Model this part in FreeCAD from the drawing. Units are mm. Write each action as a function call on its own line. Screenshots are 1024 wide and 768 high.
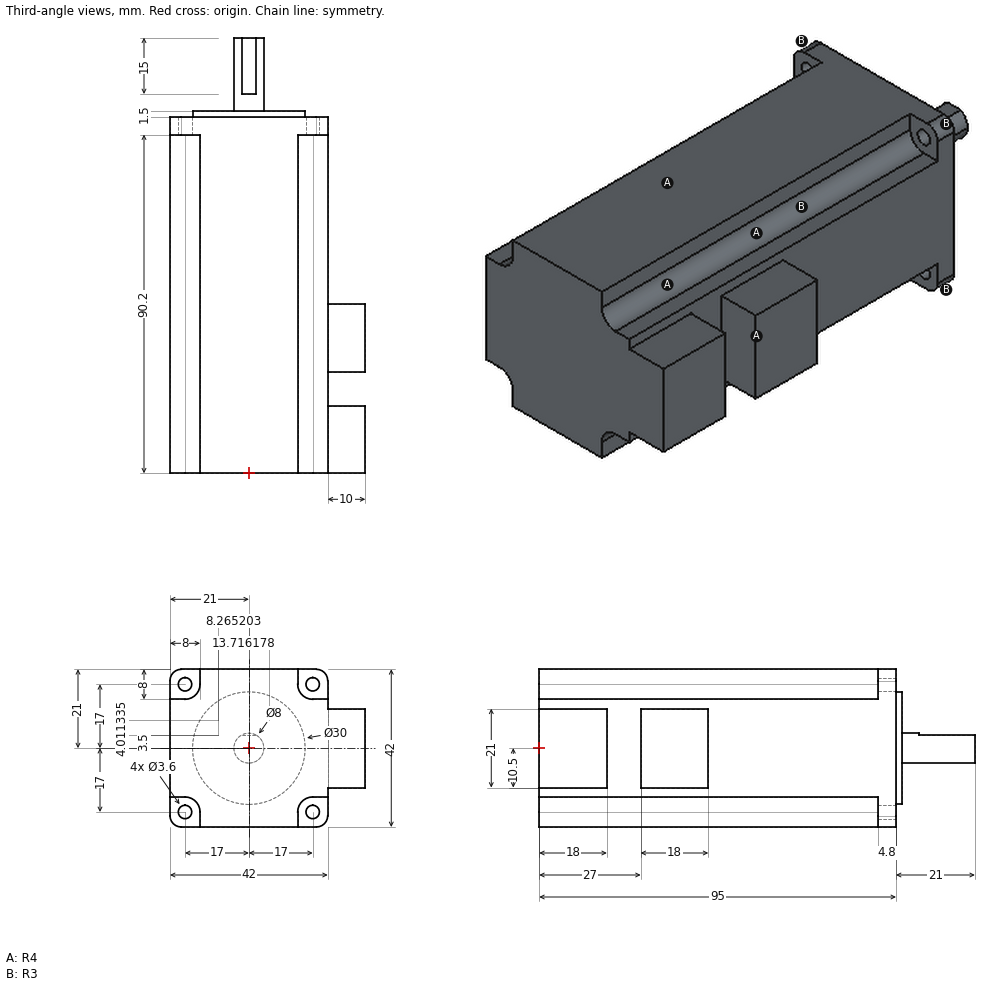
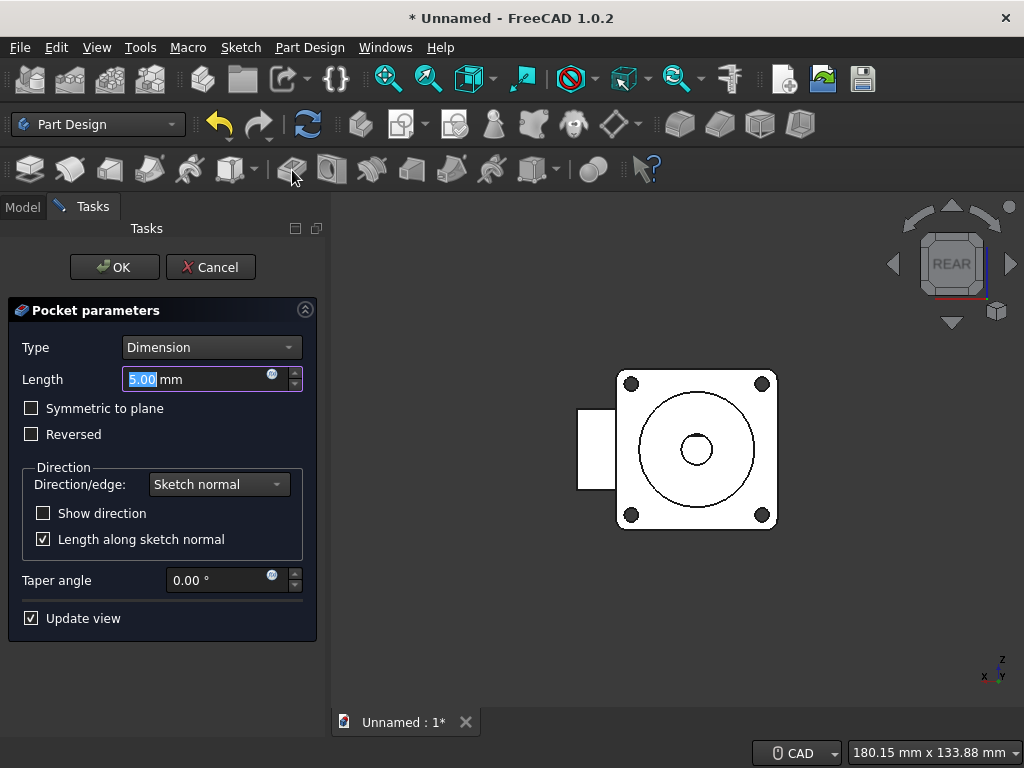
text(15)
key(Tab)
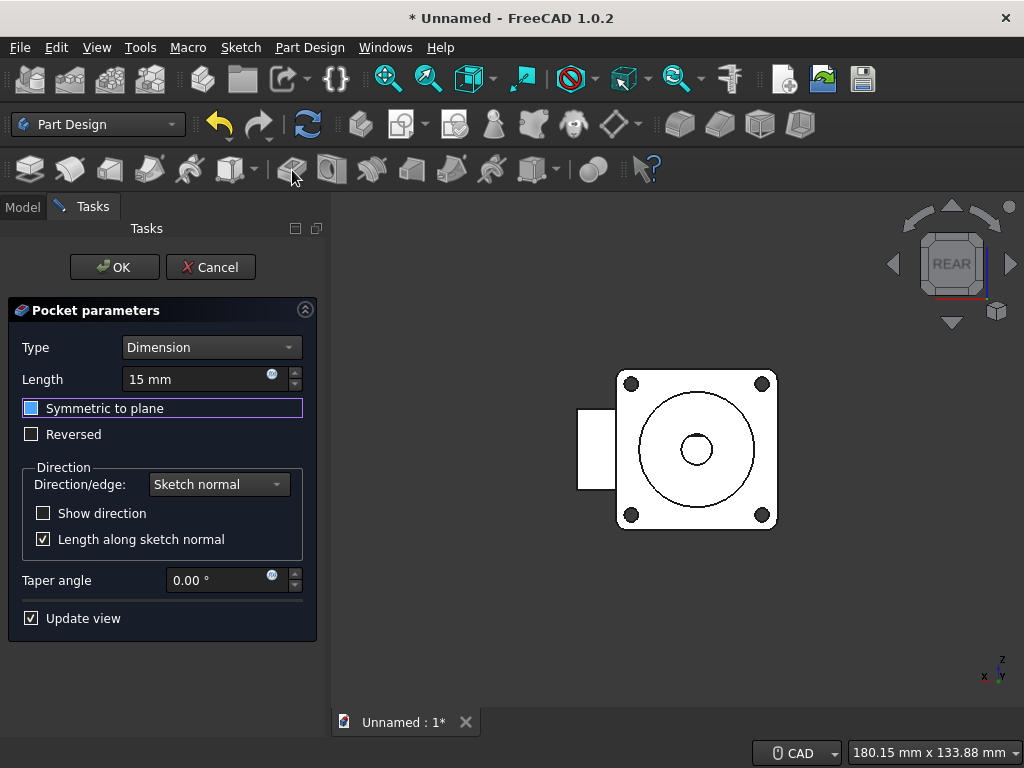
click(115, 267)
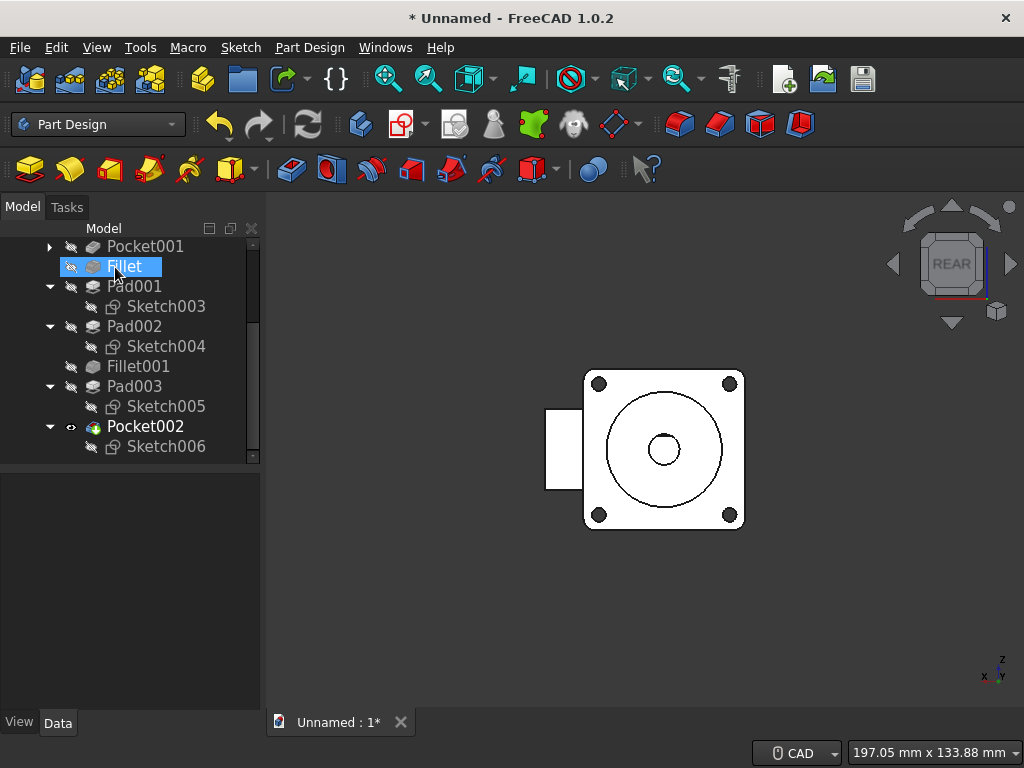
key(0)